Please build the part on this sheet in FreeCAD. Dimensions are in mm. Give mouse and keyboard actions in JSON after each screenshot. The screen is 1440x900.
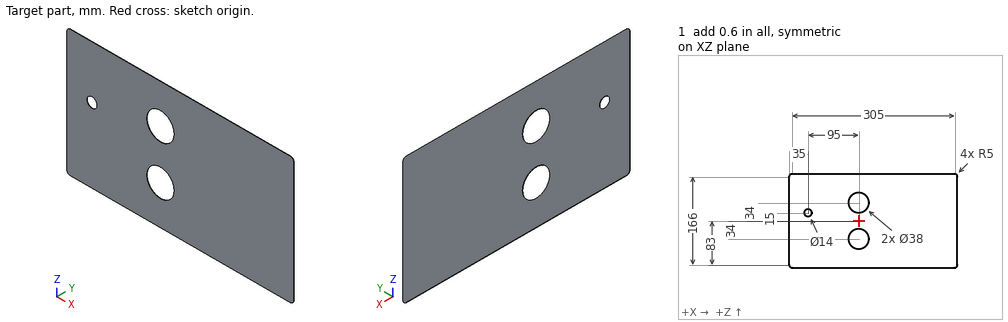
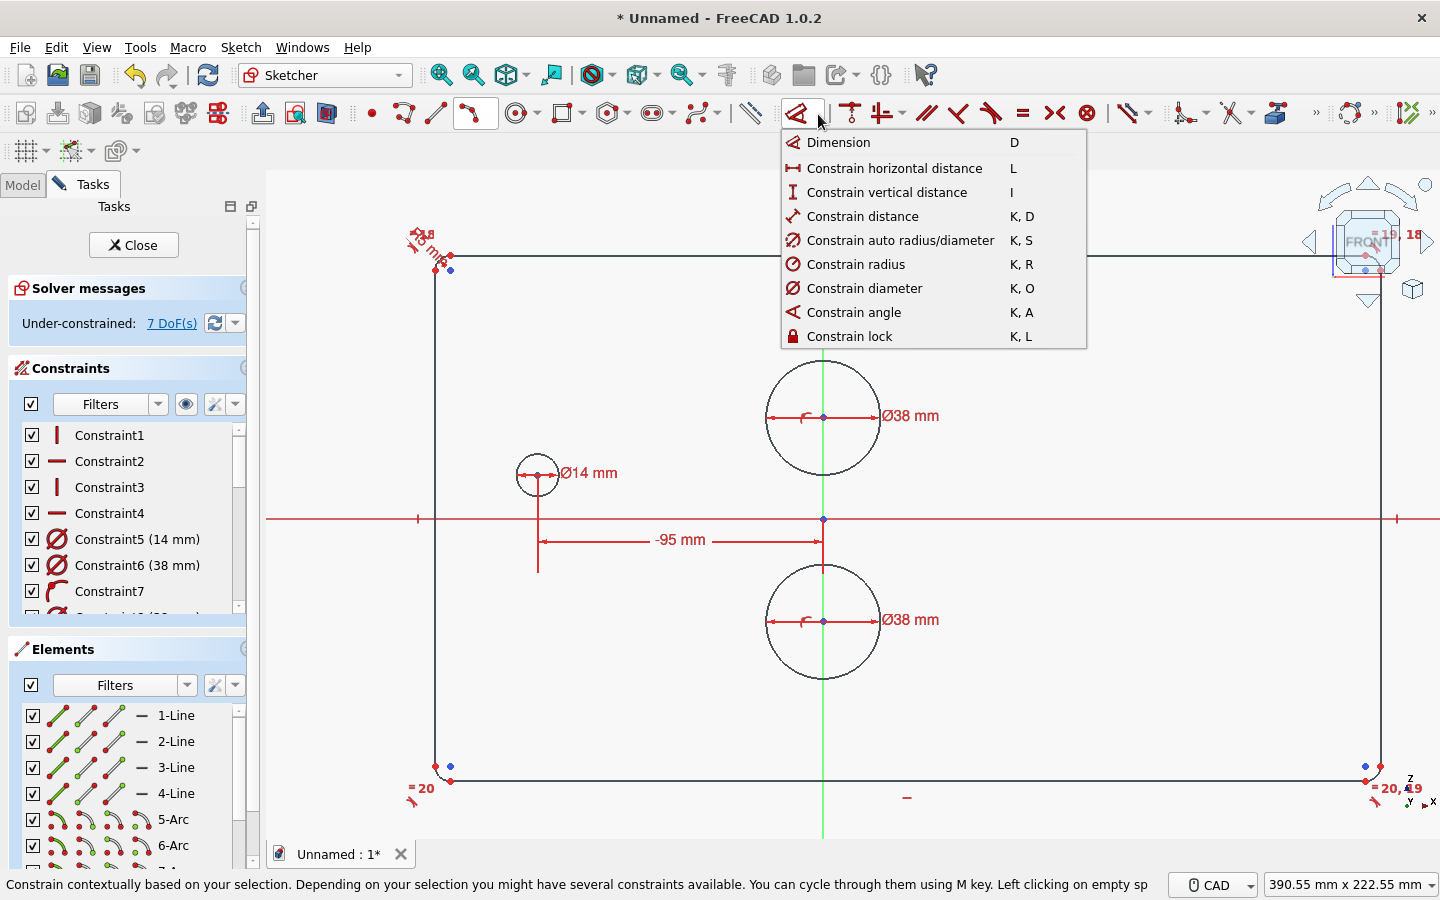
{"action": "left_click", "coordinate": [934, 192]}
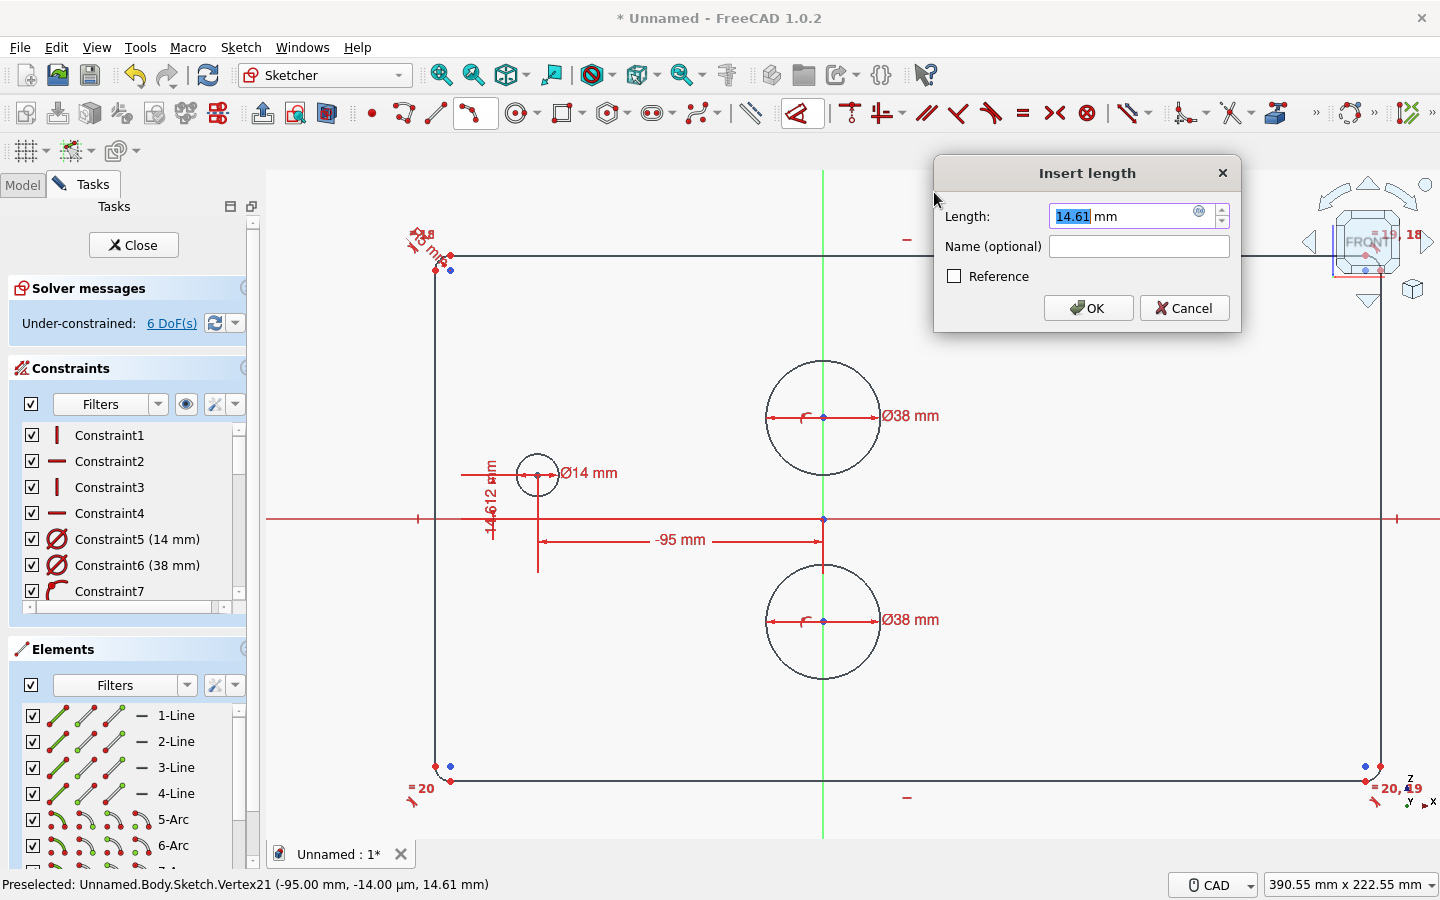
{"action": "type", "text": "15"}
{"action": "key", "text": "Return"}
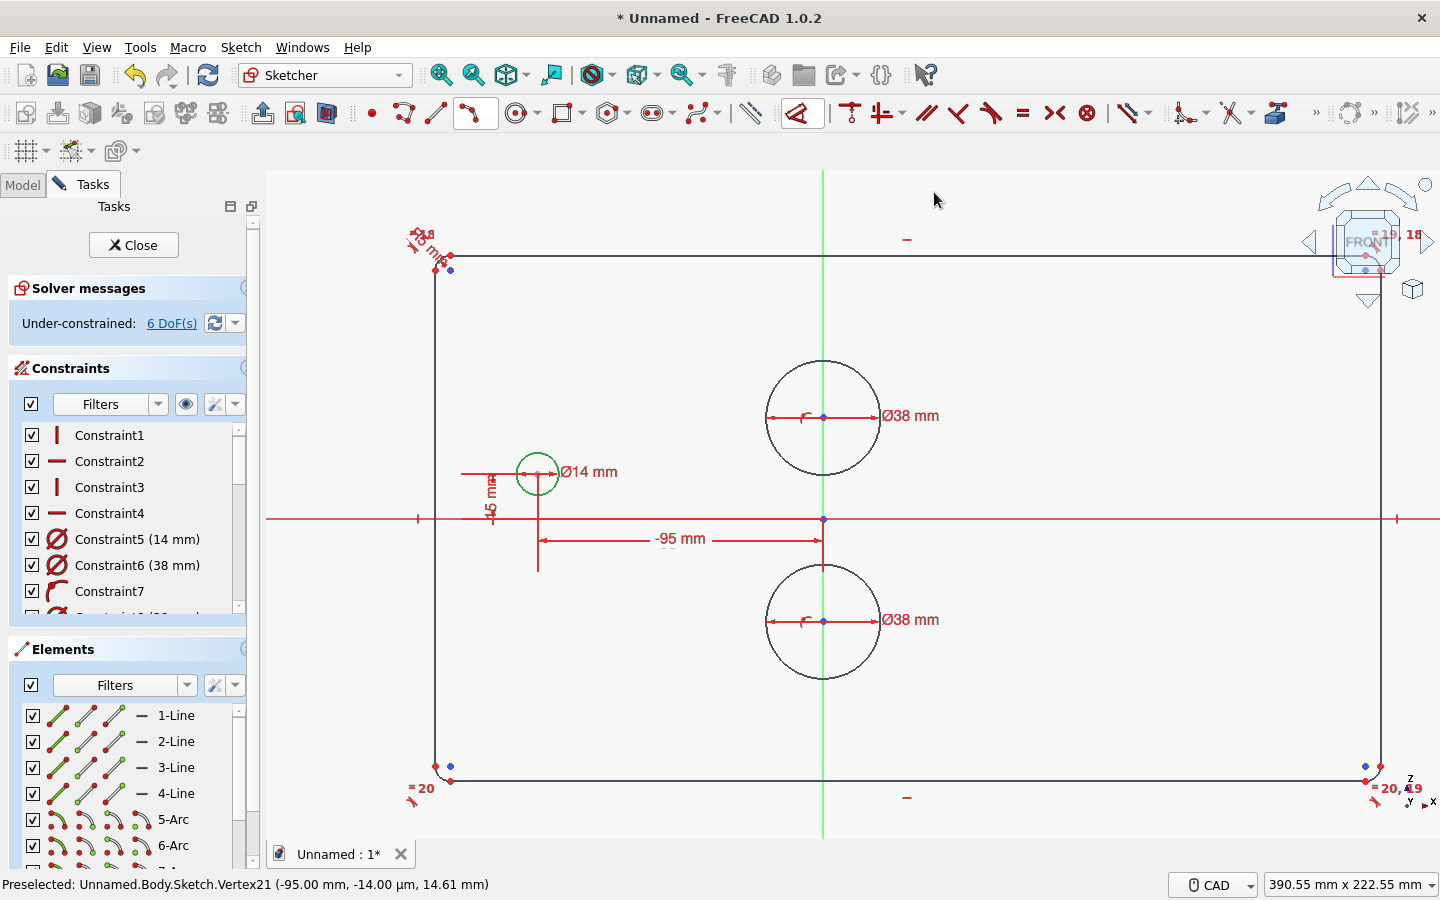
{"action": "left_click", "coordinate": [823, 418]}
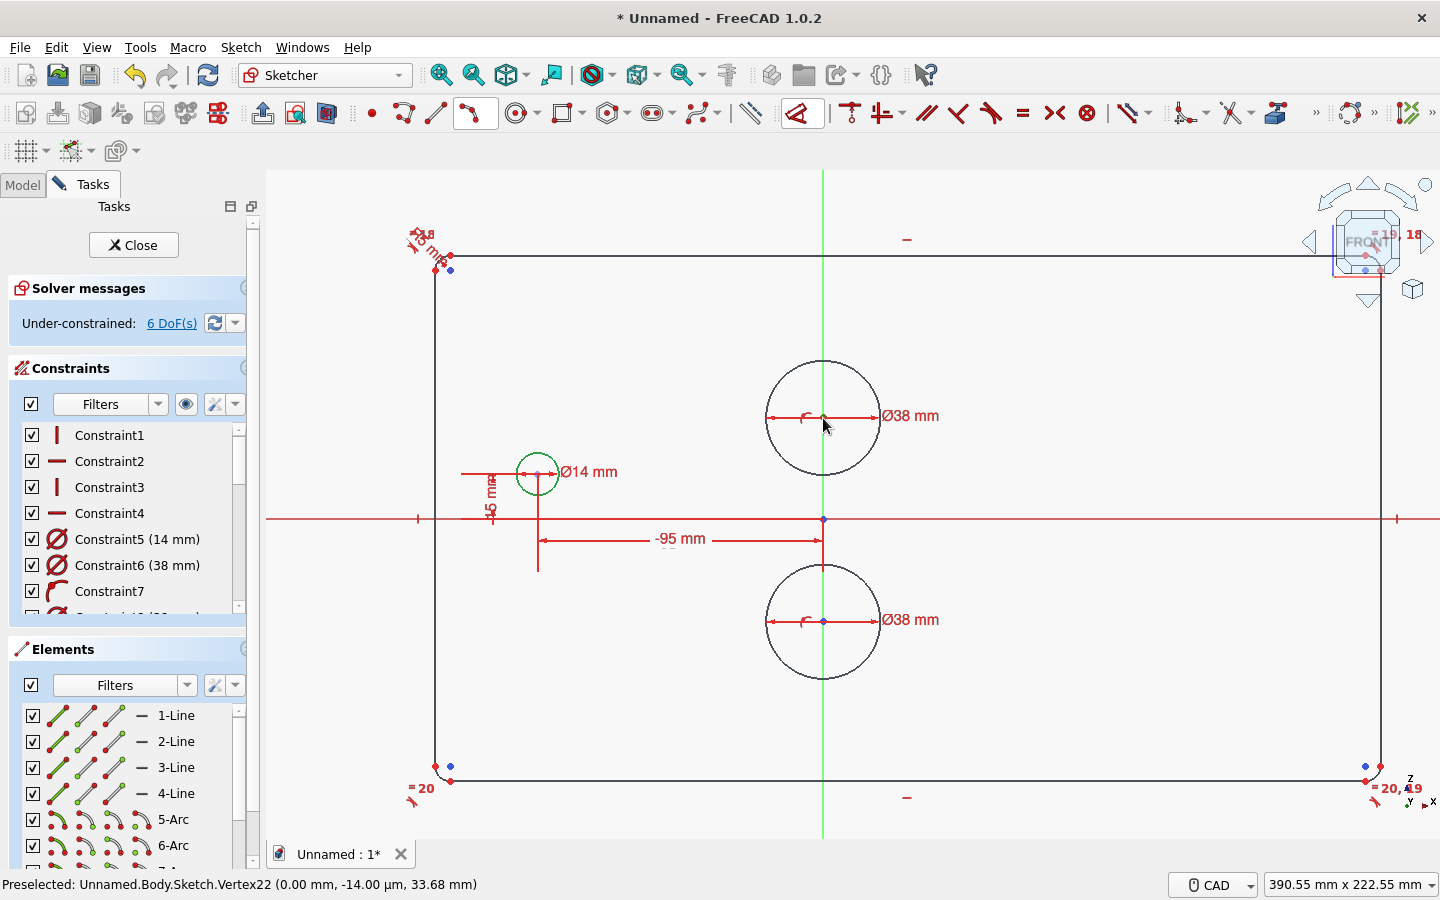
{"action": "left_click", "coordinate": [818, 114]}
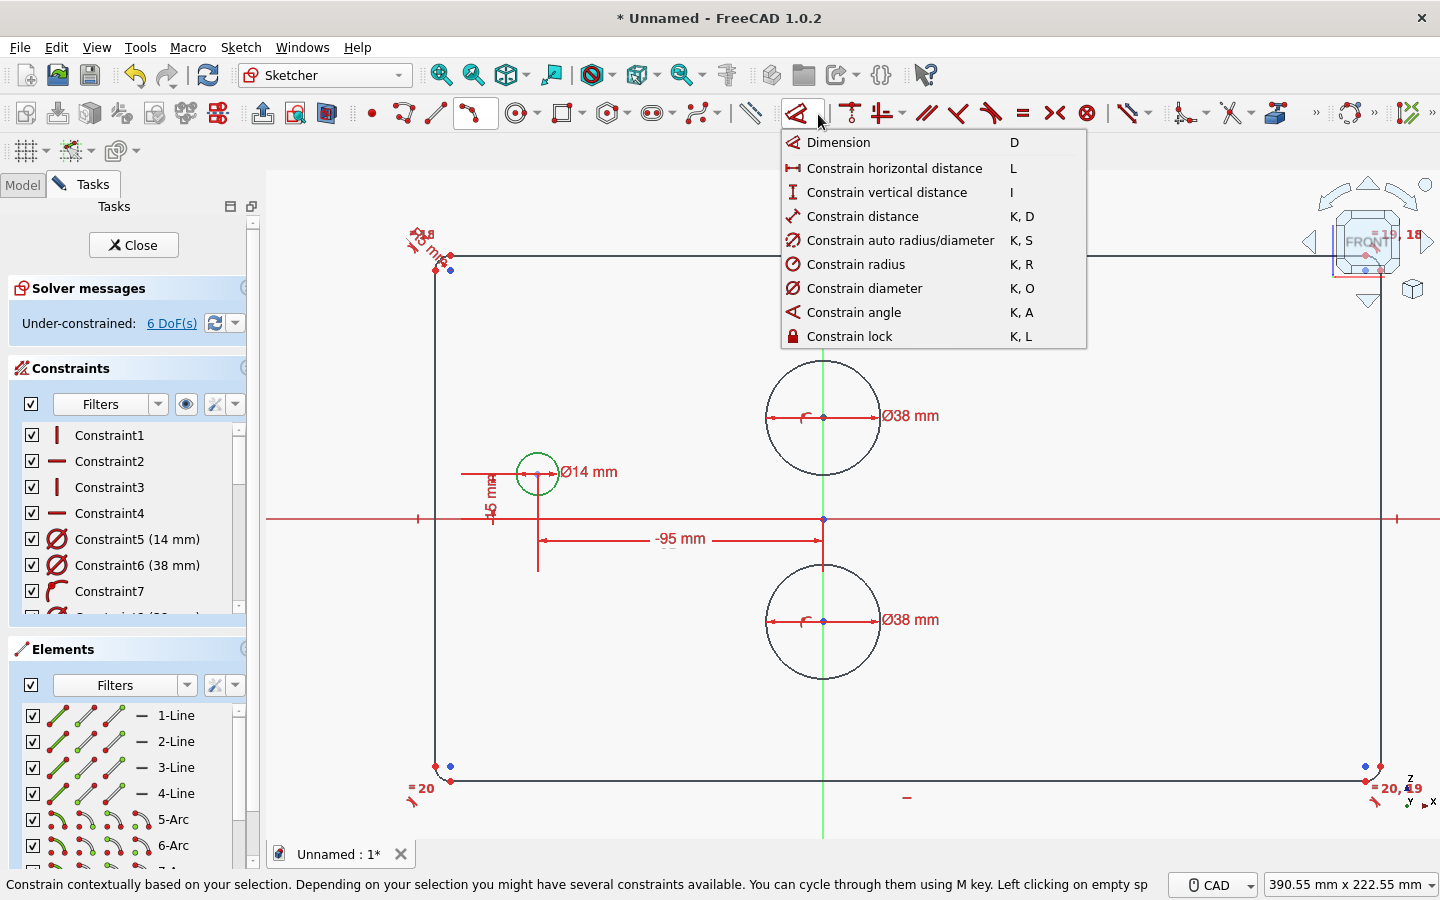
{"action": "left_click", "coordinate": [934, 192]}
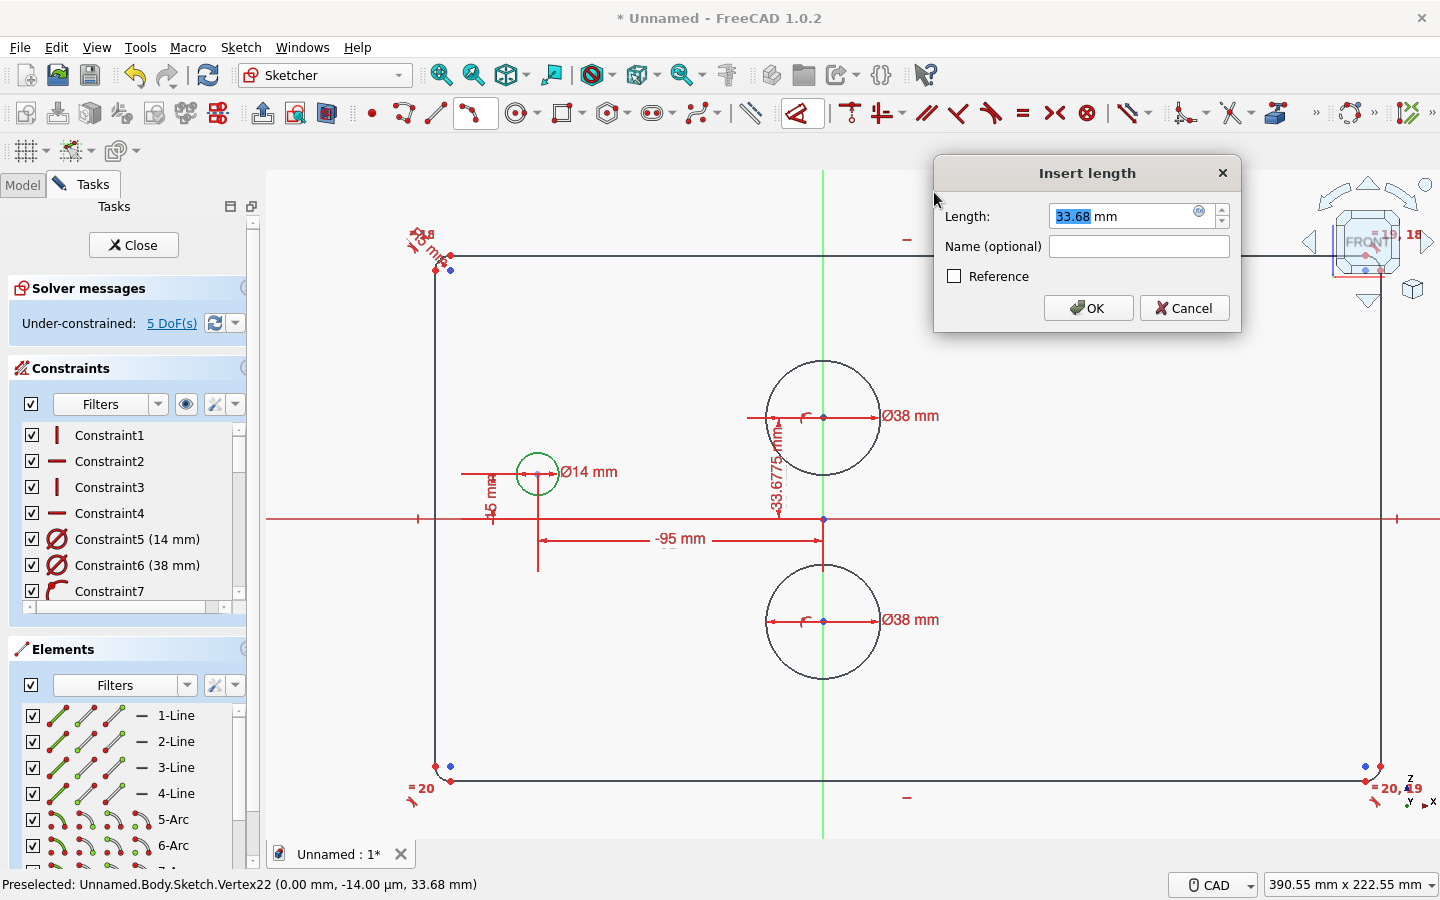
{"action": "type", "text": "34"}
{"action": "key", "text": "Return"}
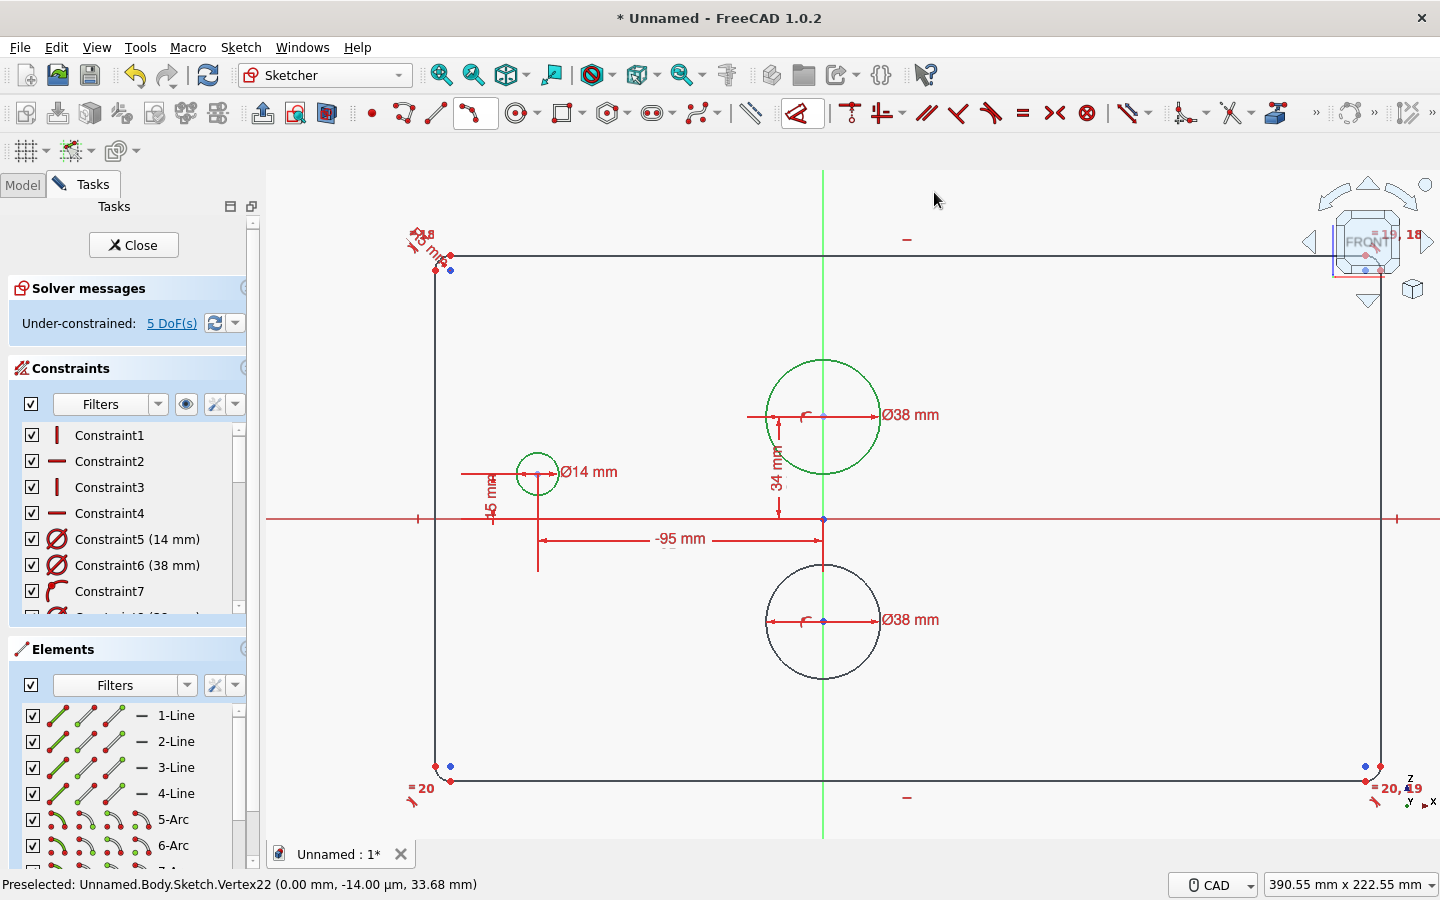
{"action": "left_click", "coordinate": [823, 622]}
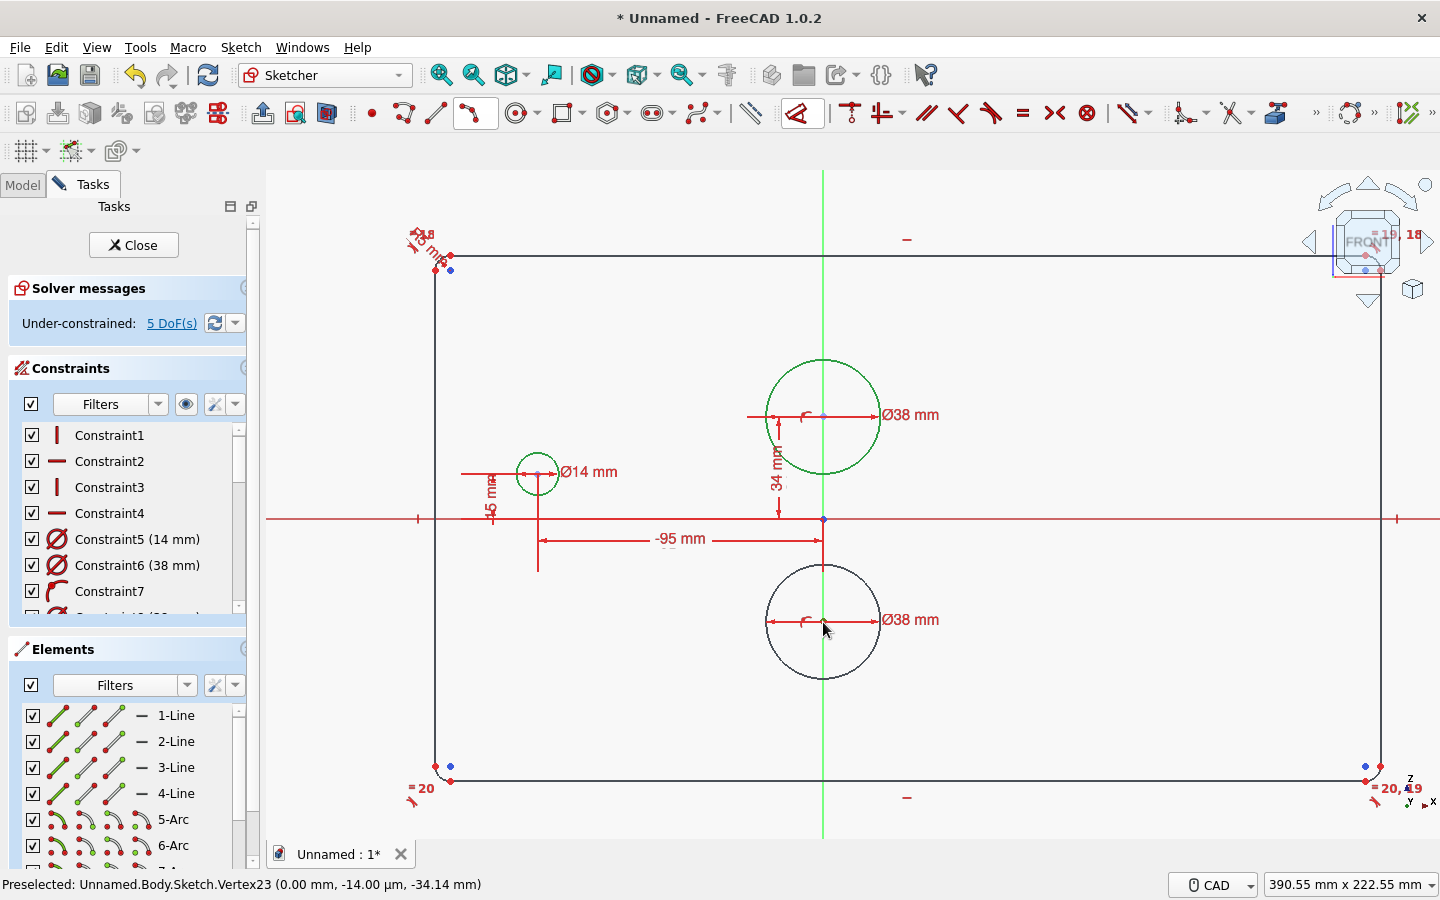
{"action": "left_click", "coordinate": [818, 114]}